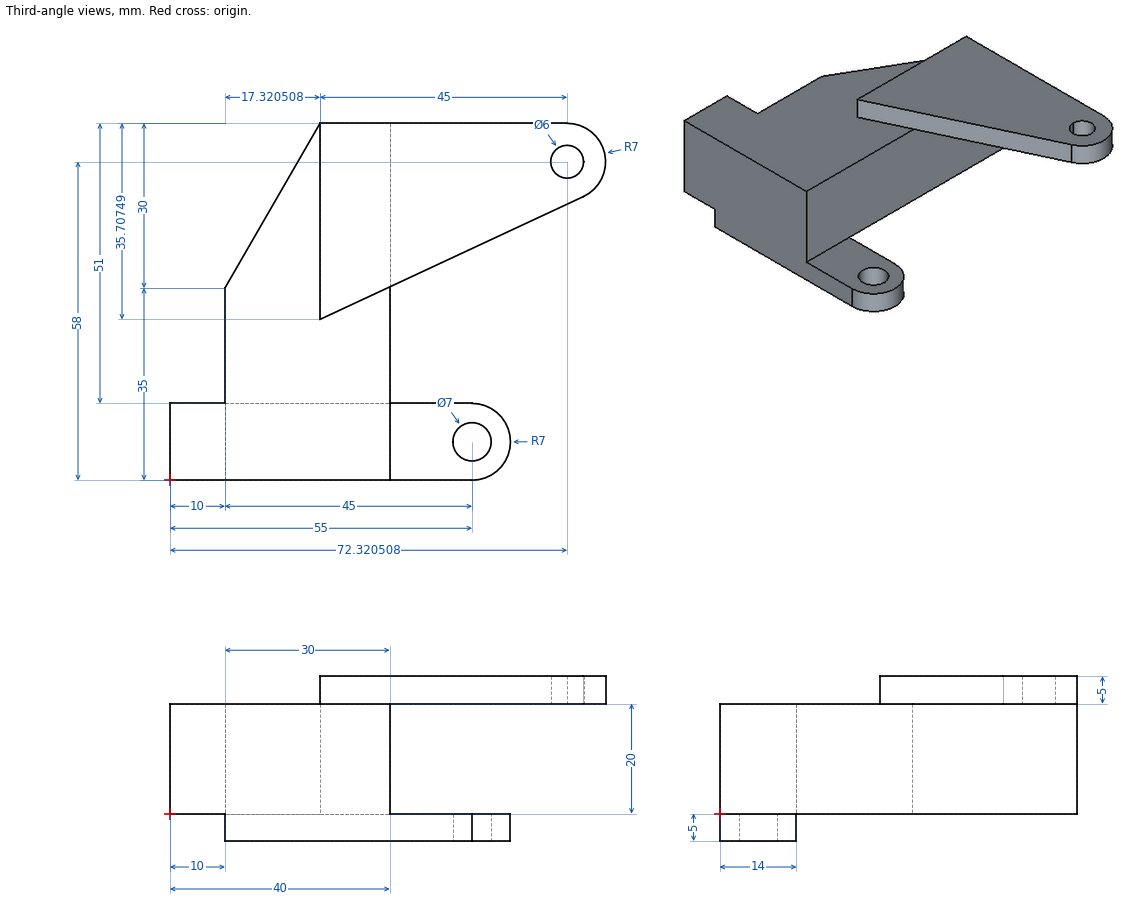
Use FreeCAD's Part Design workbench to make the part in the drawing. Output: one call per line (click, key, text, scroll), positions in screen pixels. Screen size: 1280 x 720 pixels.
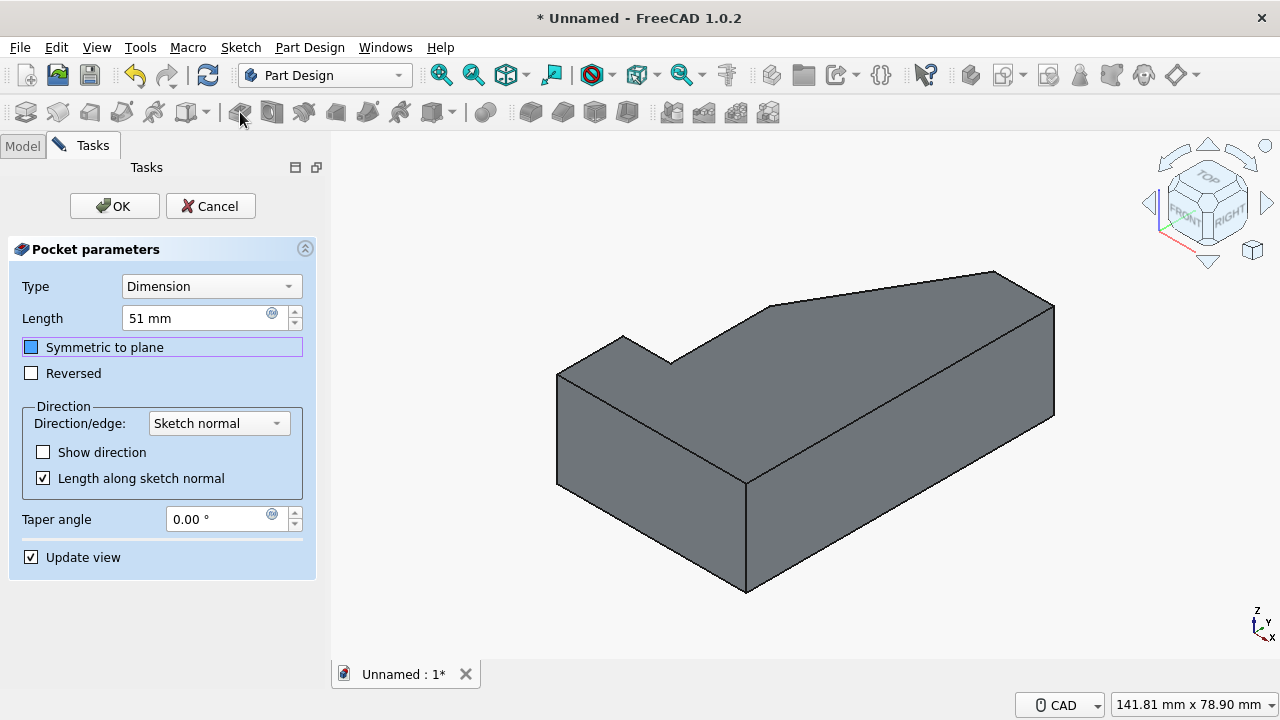
click(115, 206)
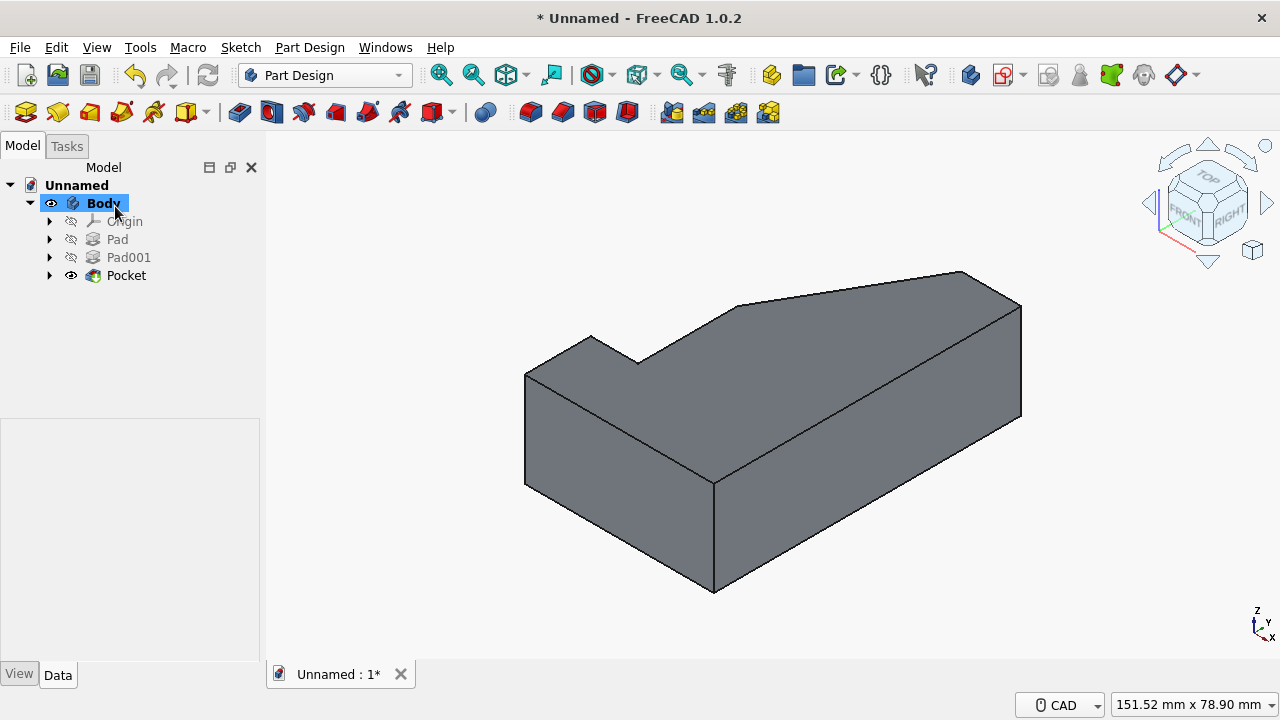
click(800, 355)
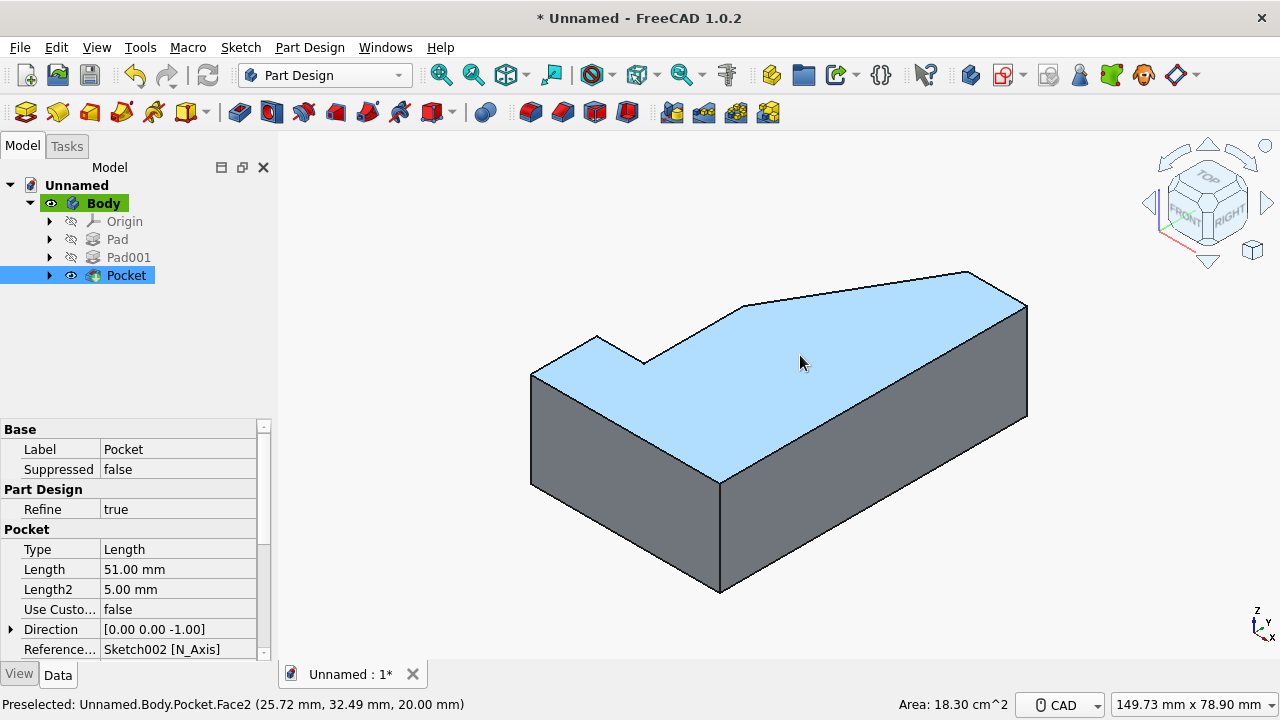
click(1004, 76)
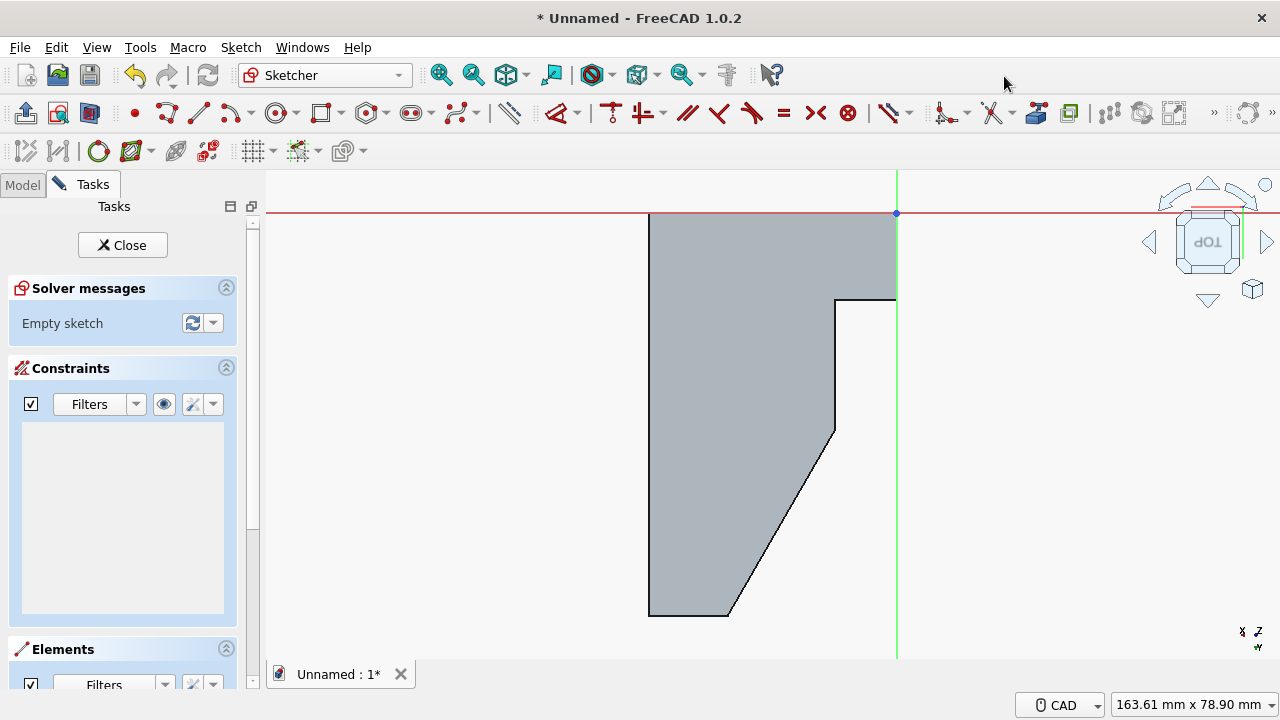
scroll(943, 415, down, 1)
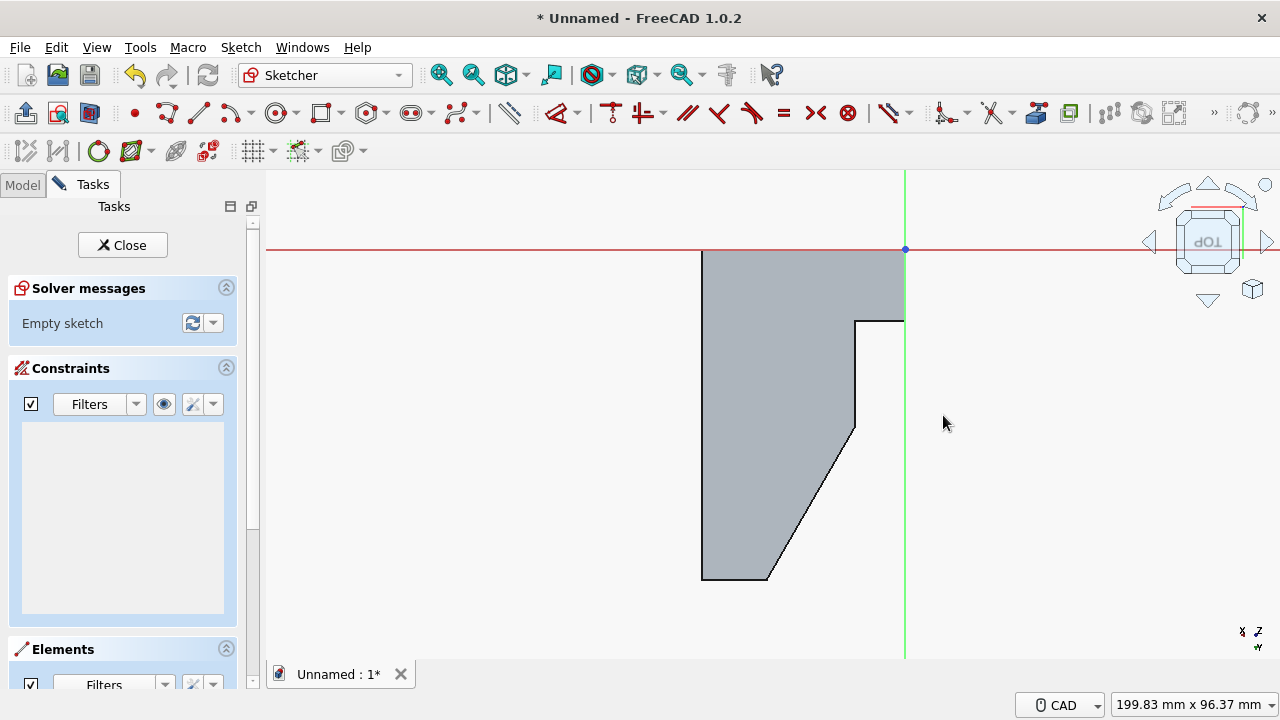
click(168, 114)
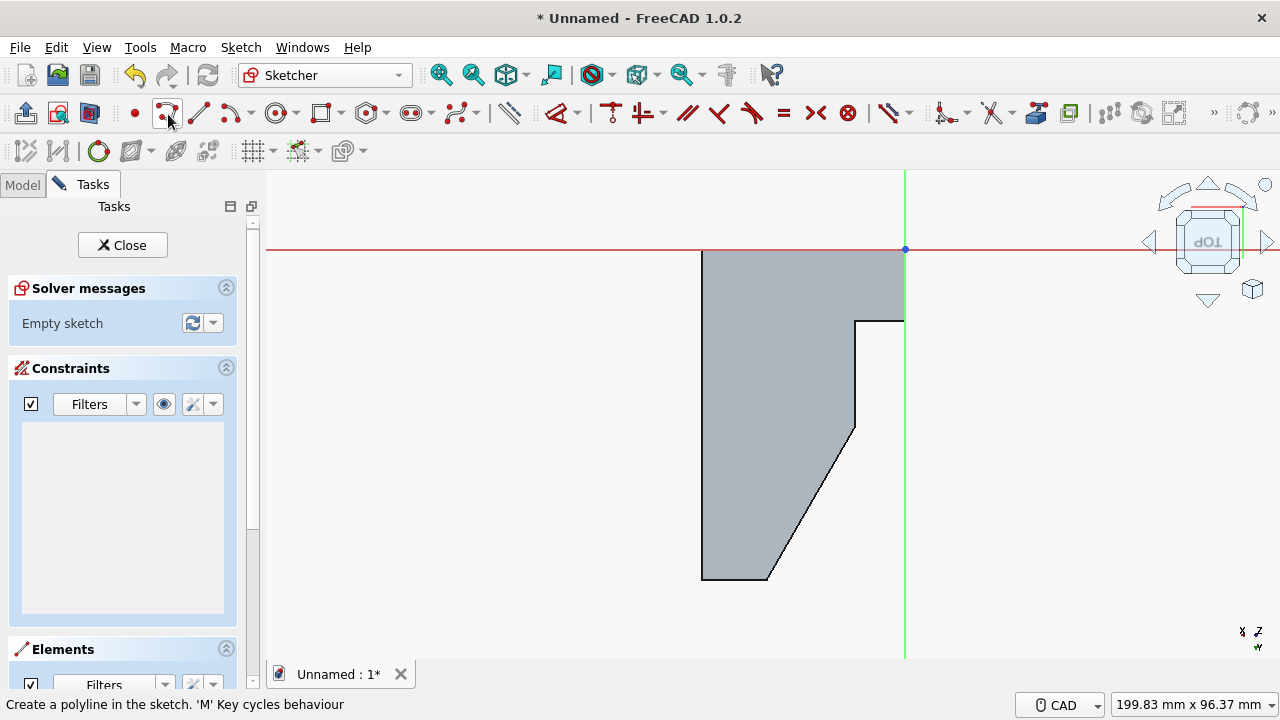
click(538, 580)
click(767, 580)
click(767, 398)
click(523, 512)
right_click(523, 512)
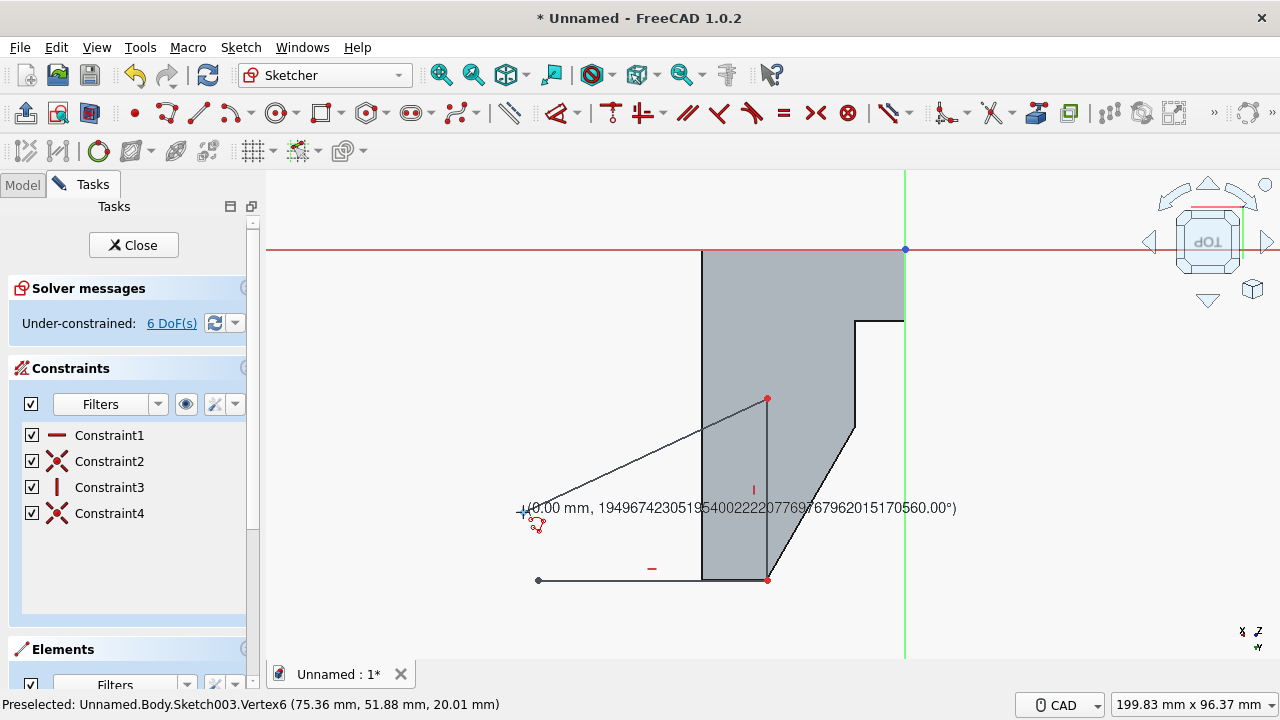
key(g)
key(3)
key(a)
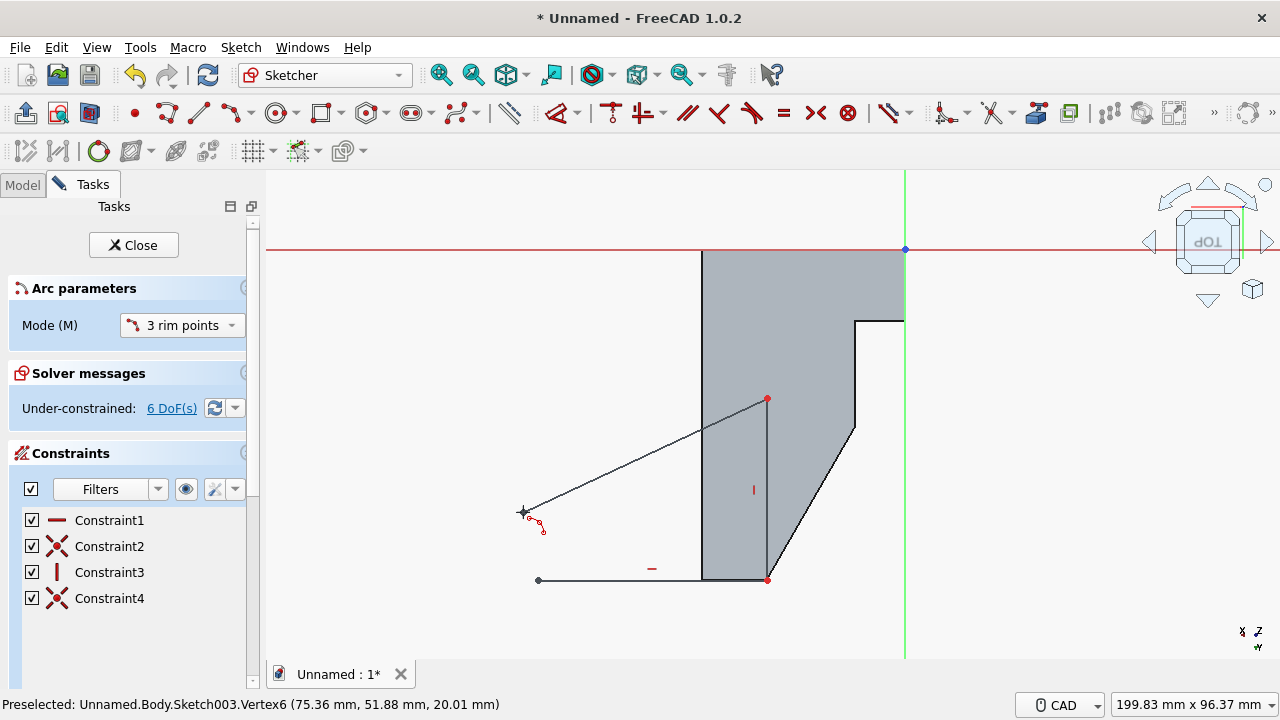
click(523, 513)
click(538, 581)
click(504, 552)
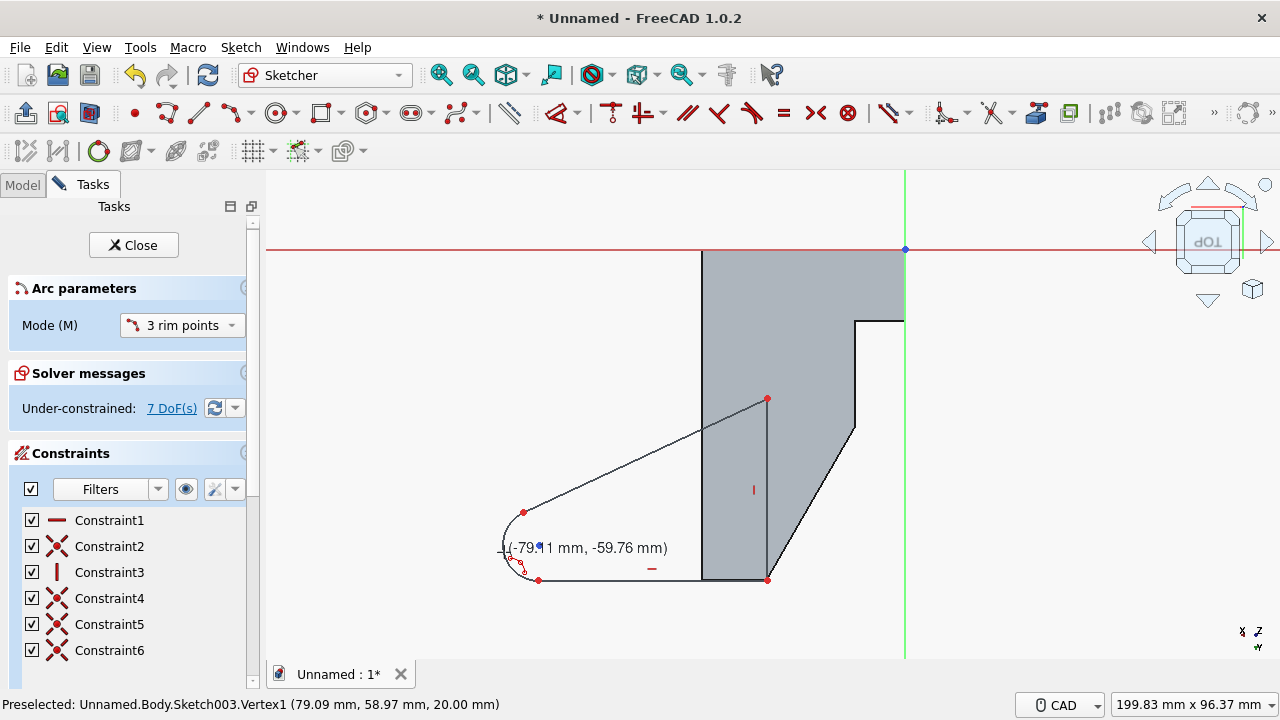
key(g)
key(c)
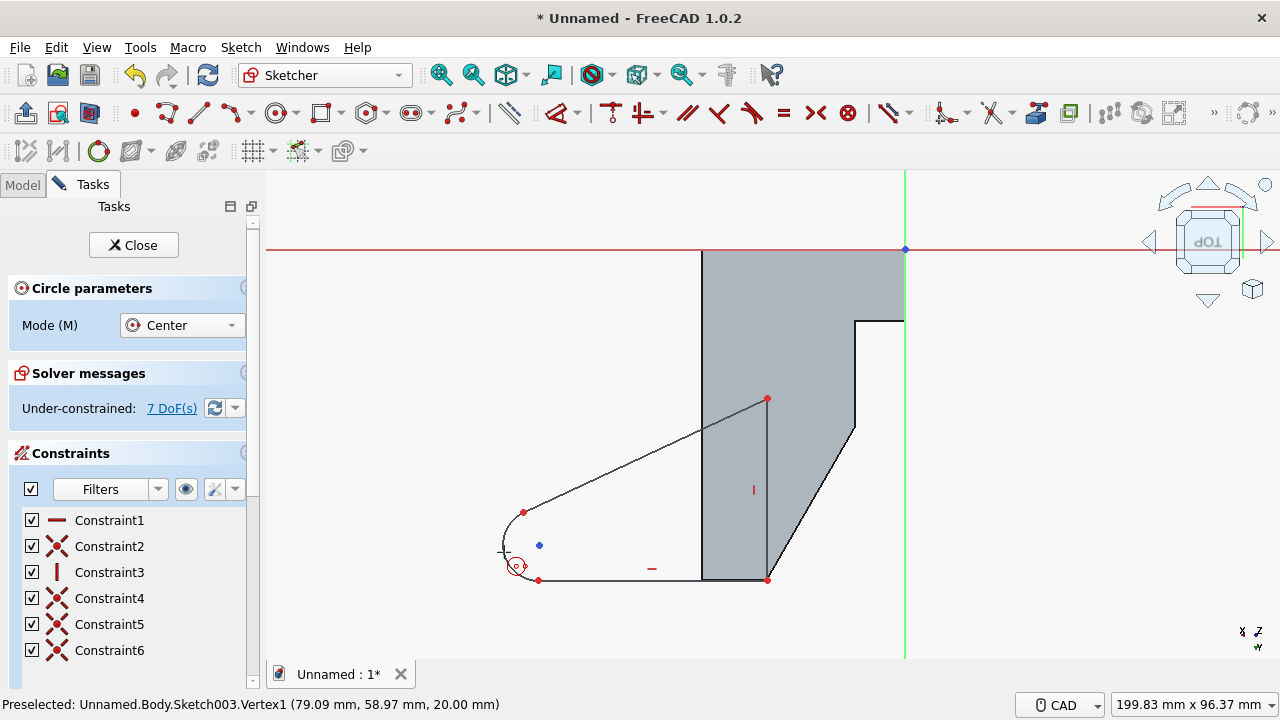
scroll(538, 544, up, 2)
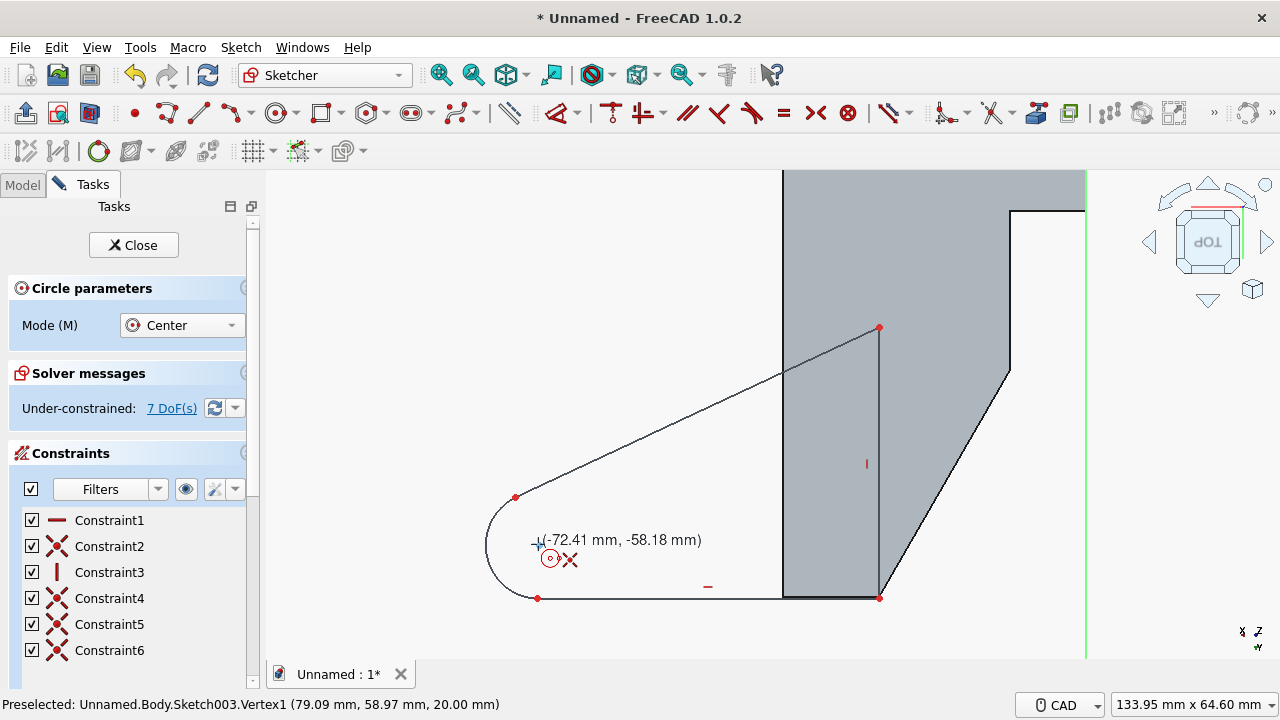
click(539, 544)
click(555, 528)
key(Escape)